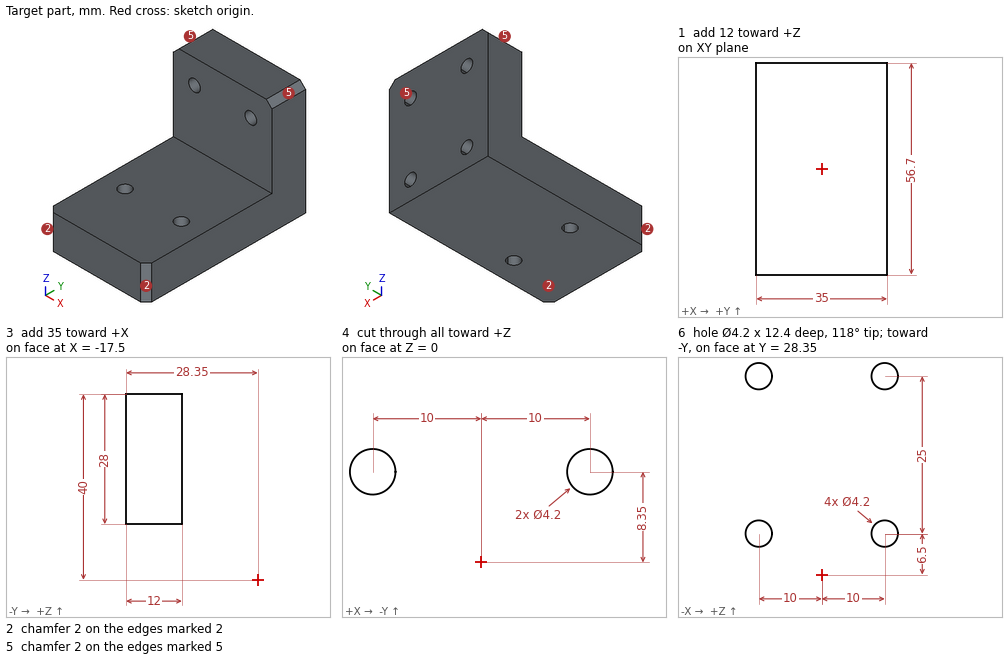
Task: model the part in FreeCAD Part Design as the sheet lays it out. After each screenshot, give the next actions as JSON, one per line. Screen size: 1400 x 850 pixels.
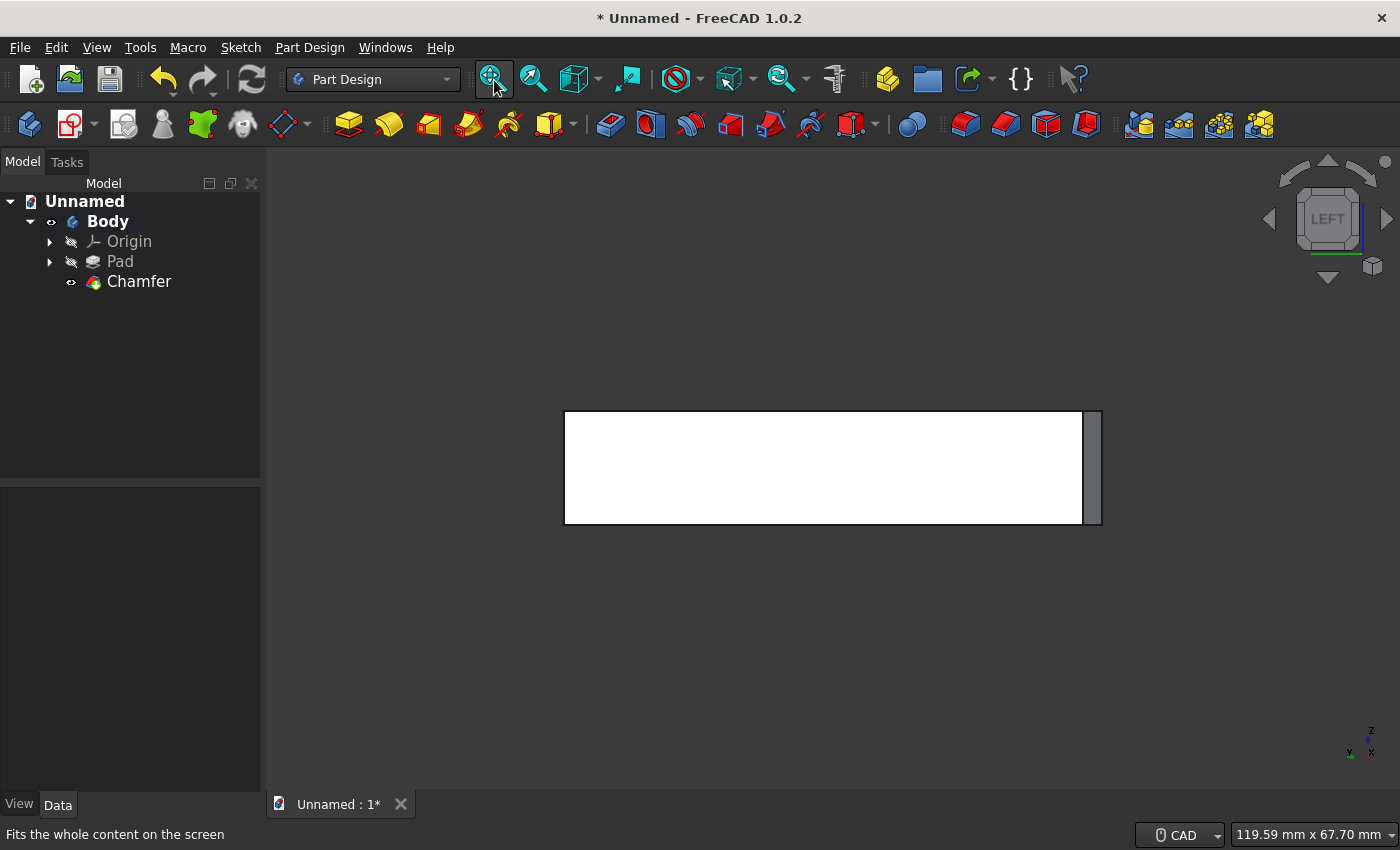
{"action": "left_click", "coordinate": [675, 467]}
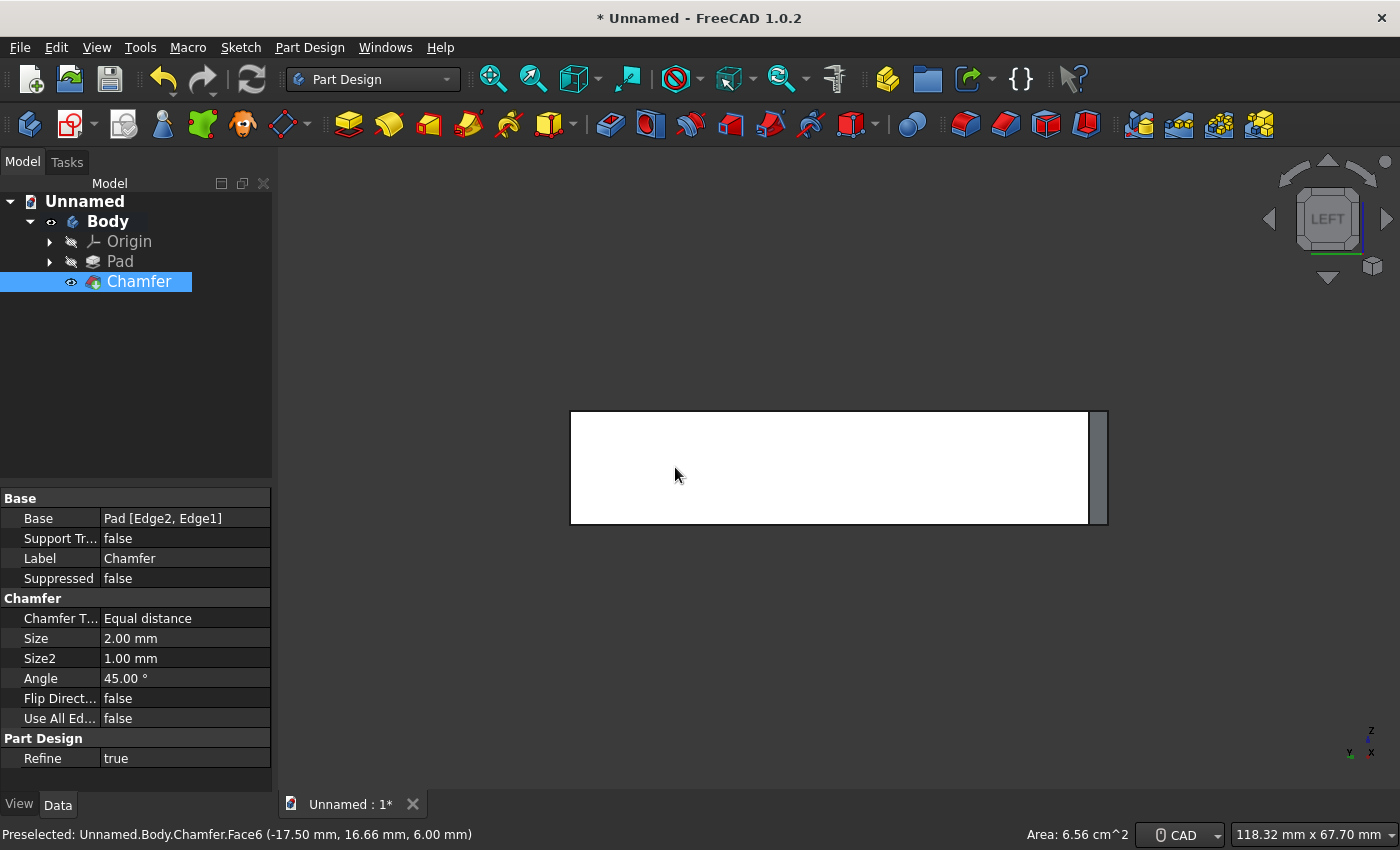
{"action": "left_click", "coordinate": [70, 124]}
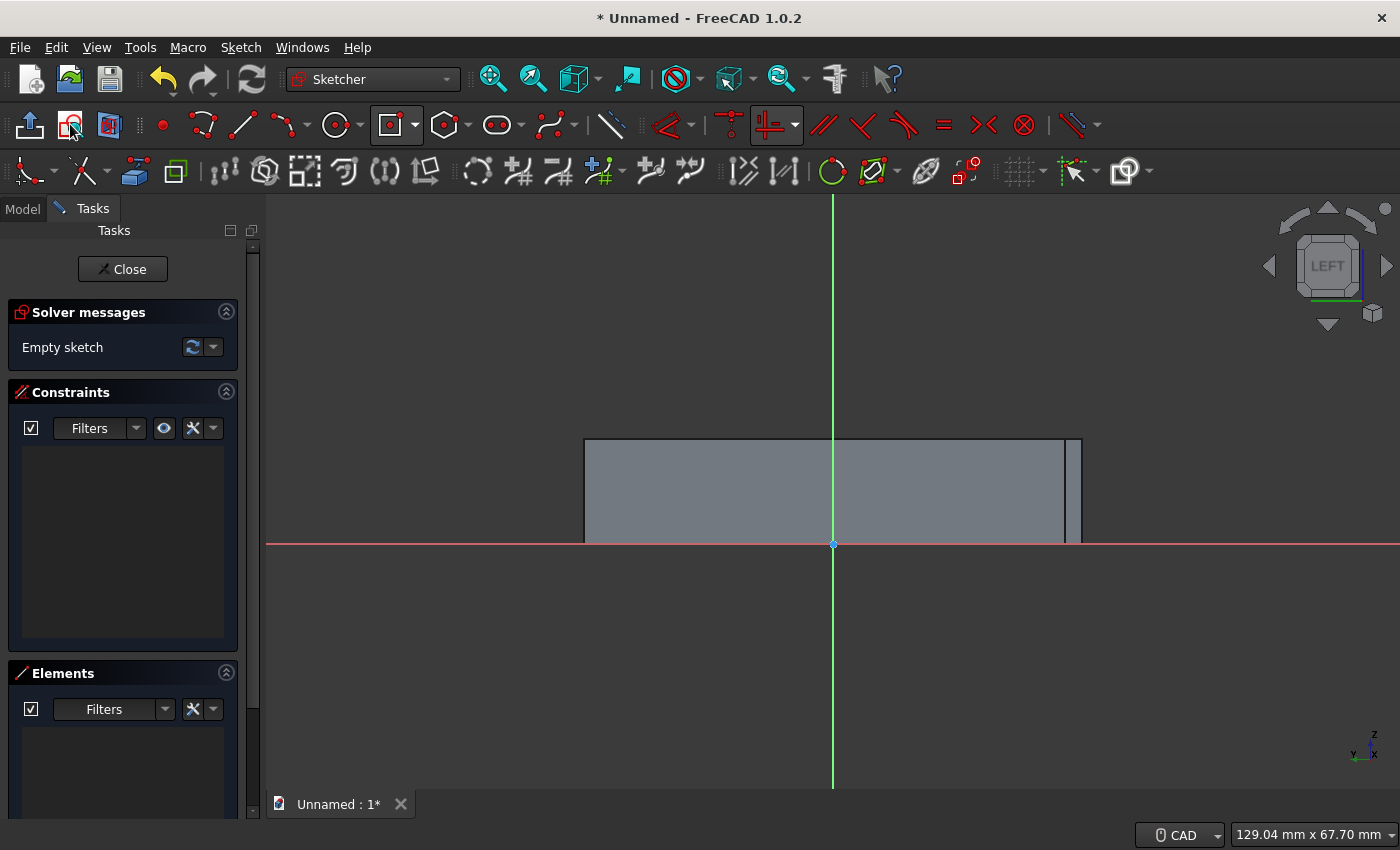
{"action": "scroll", "coordinate": [1018, 761], "scroll_direction": "down", "scroll_amount": 1}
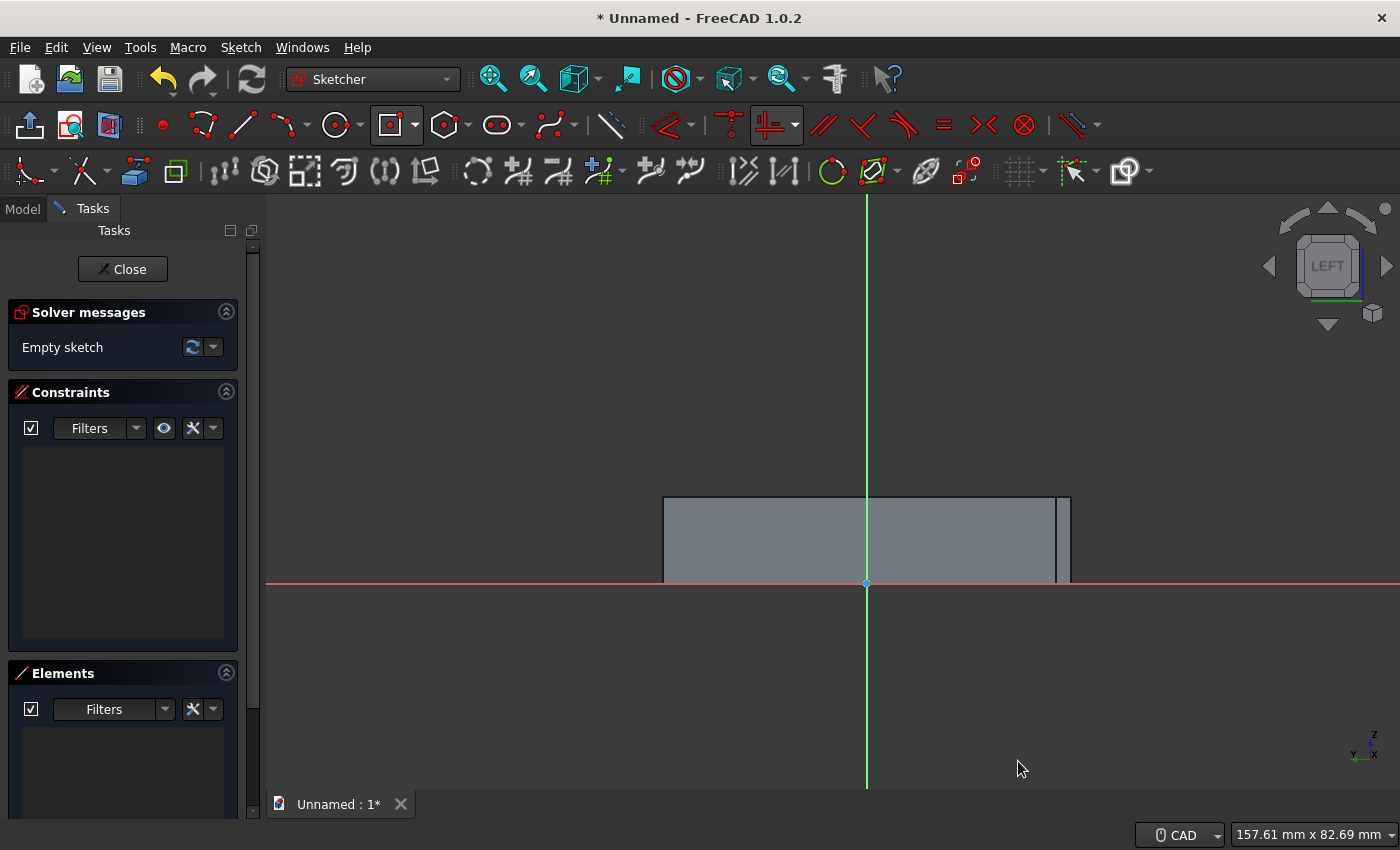
{"action": "left_click", "coordinate": [418, 126]}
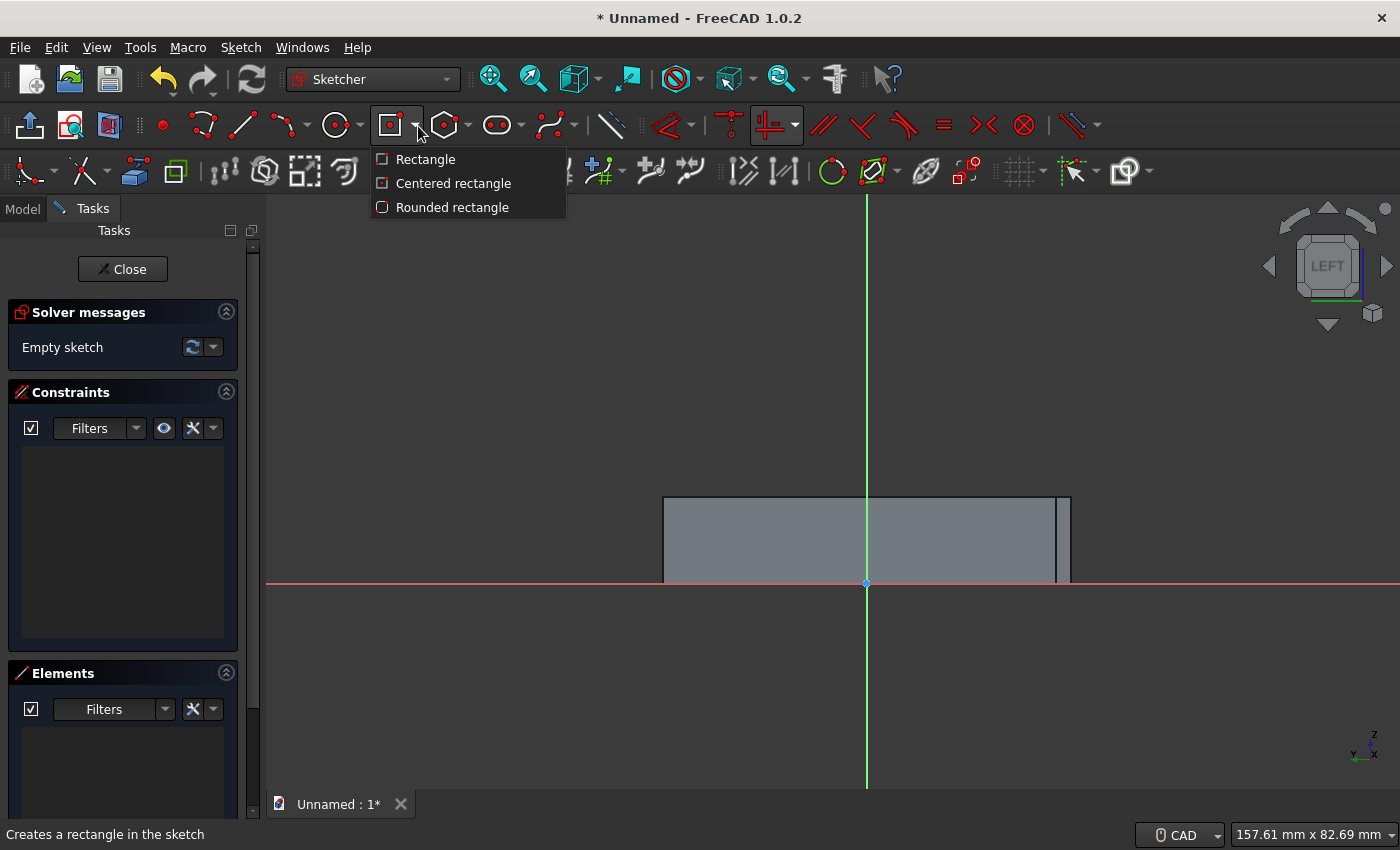
{"action": "left_click", "coordinate": [468, 159]}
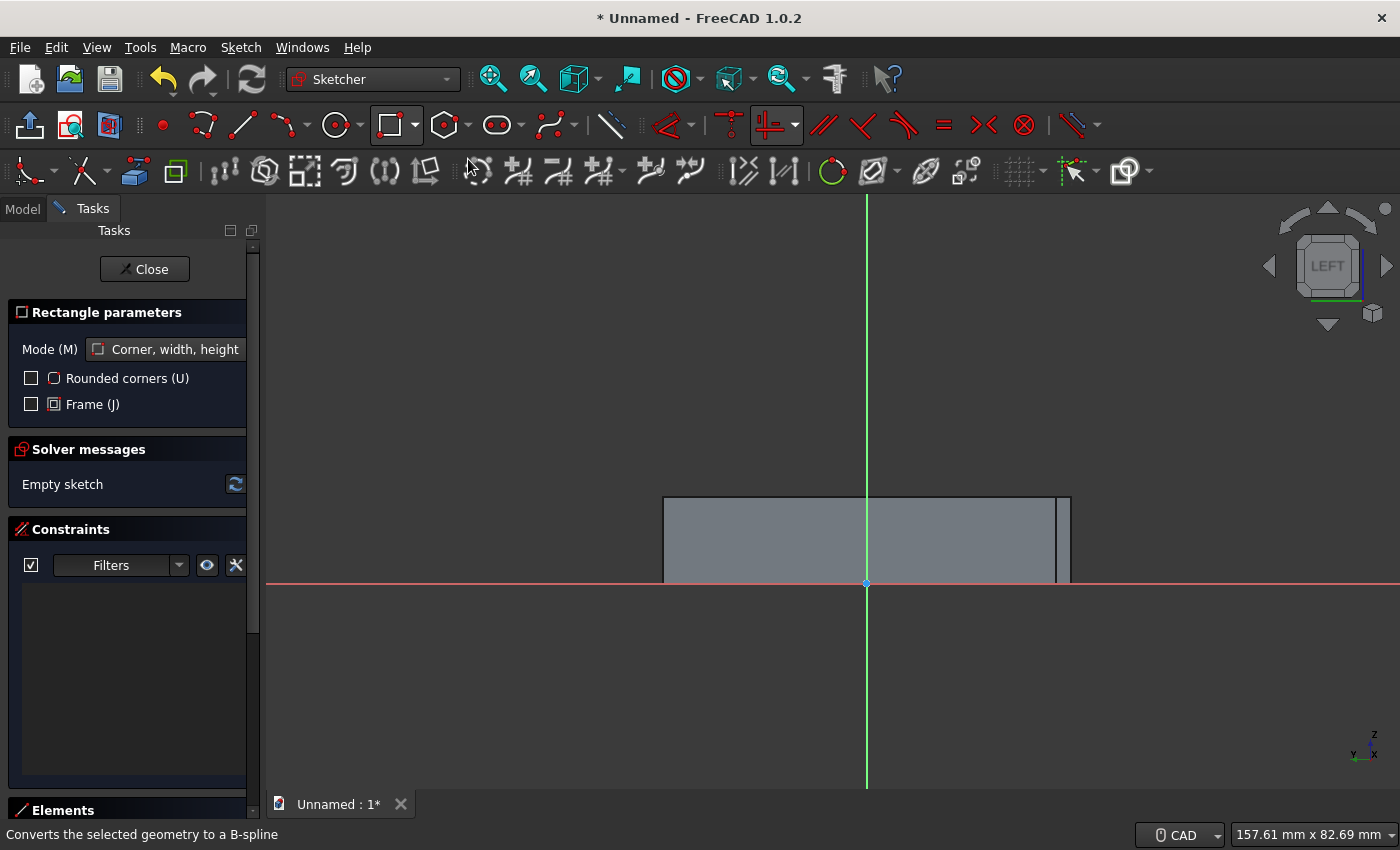
{"action": "left_click", "coordinate": [663, 296]}
{"action": "left_click", "coordinate": [749, 497]}
{"action": "key", "text": "Escape"}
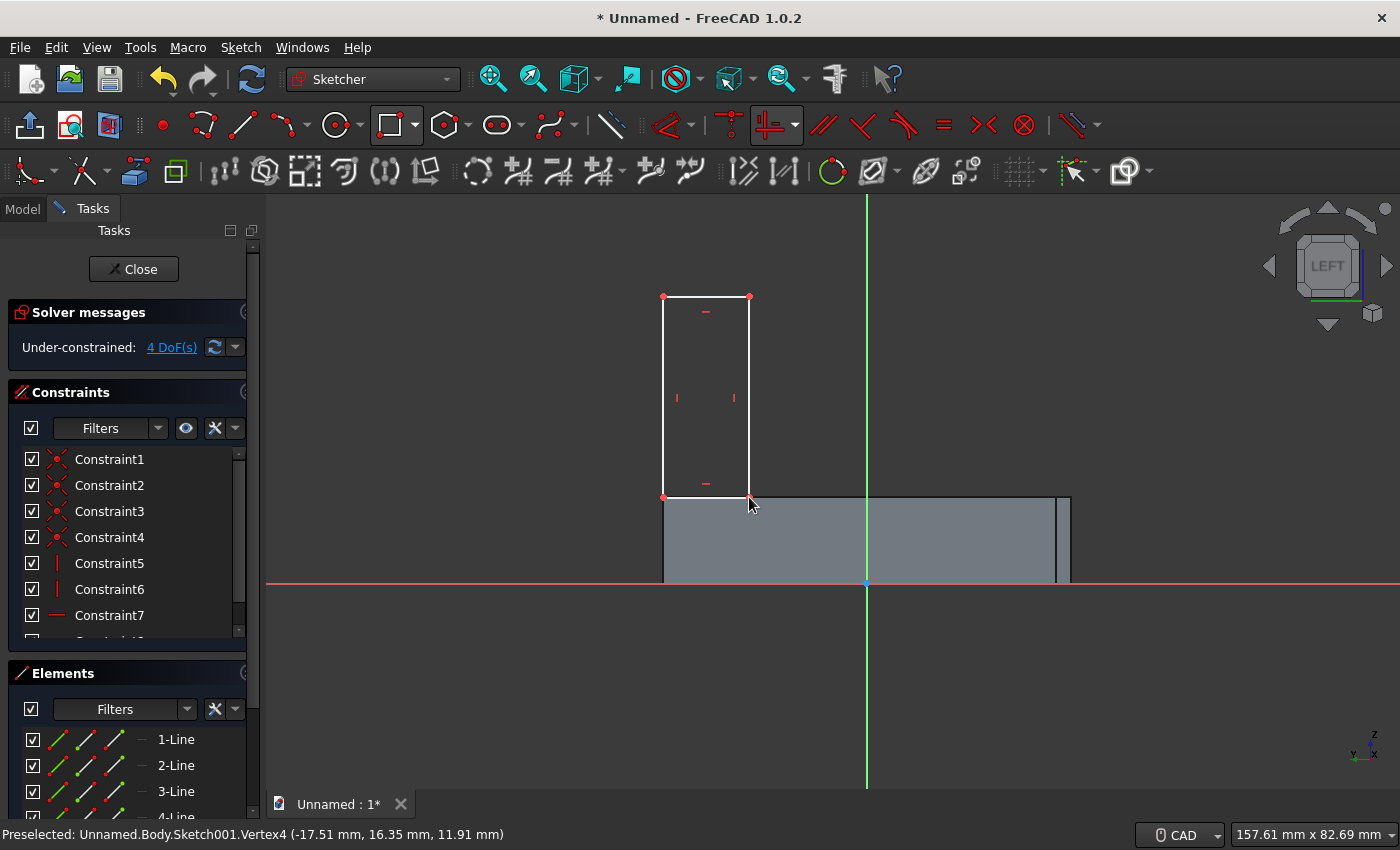
{"action": "left_click", "coordinate": [666, 126]}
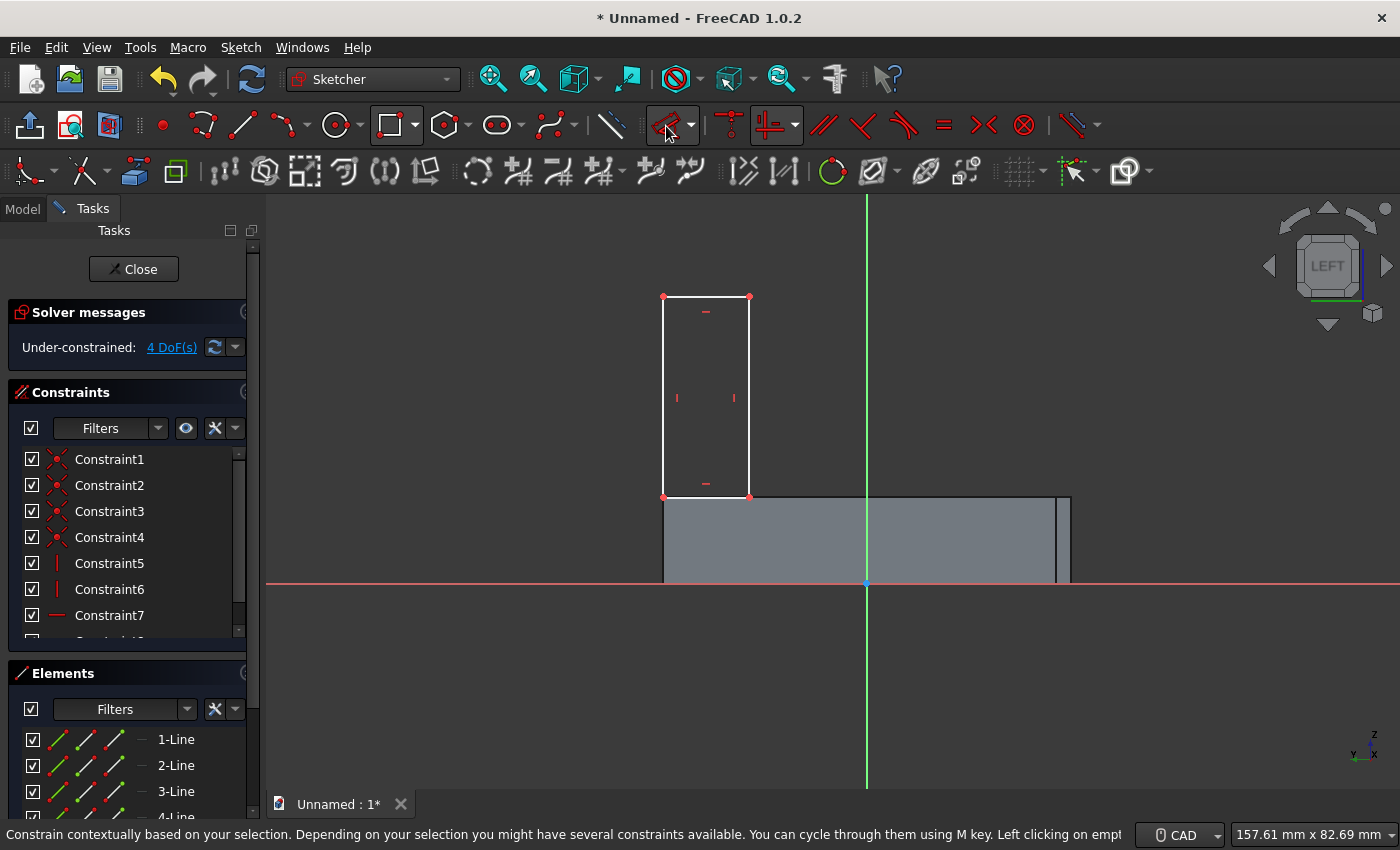
{"action": "left_click", "coordinate": [663, 357]}
{"action": "left_click", "coordinate": [629, 398]}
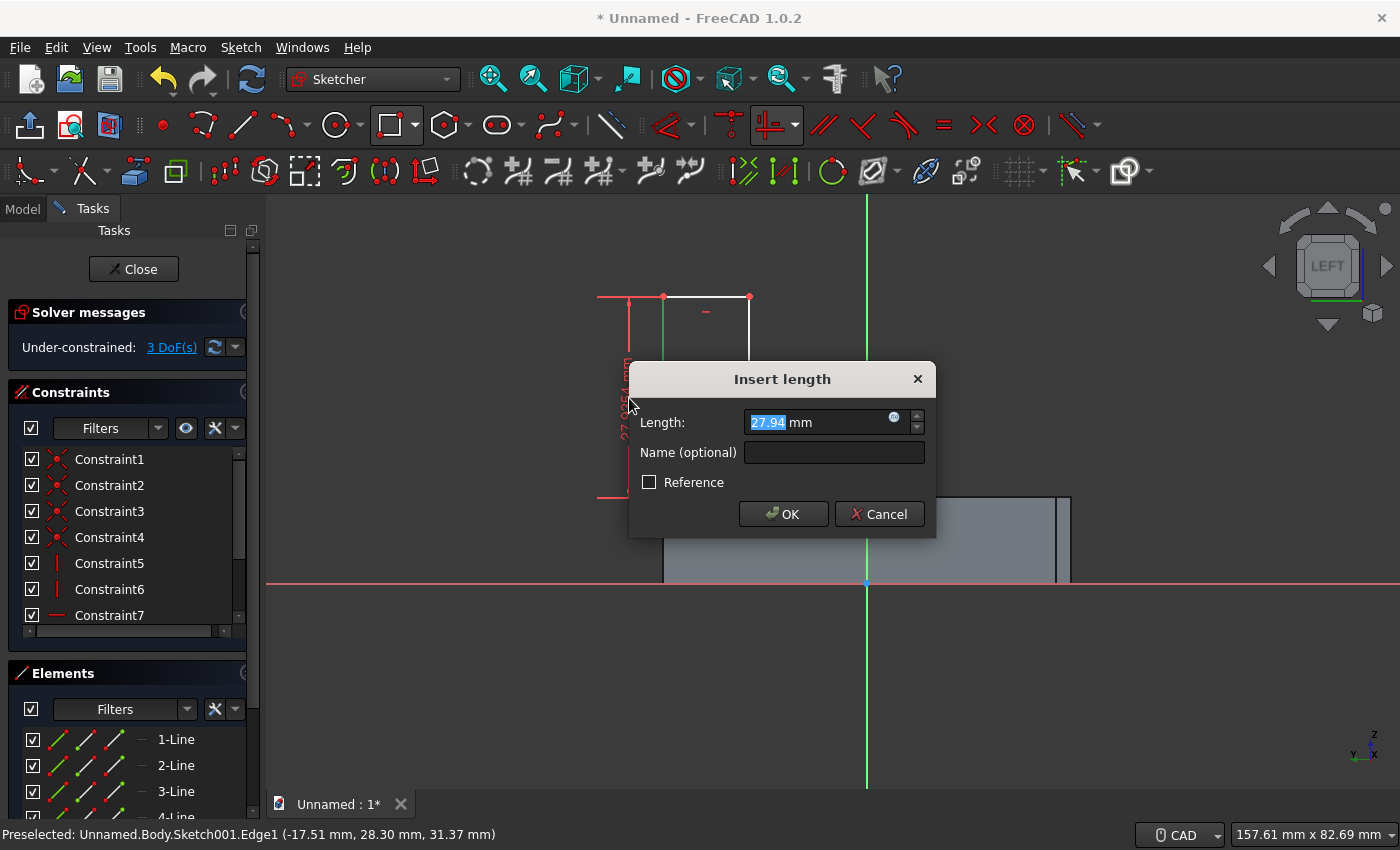
{"action": "type", "text": "28"}
{"action": "key", "text": "Return"}